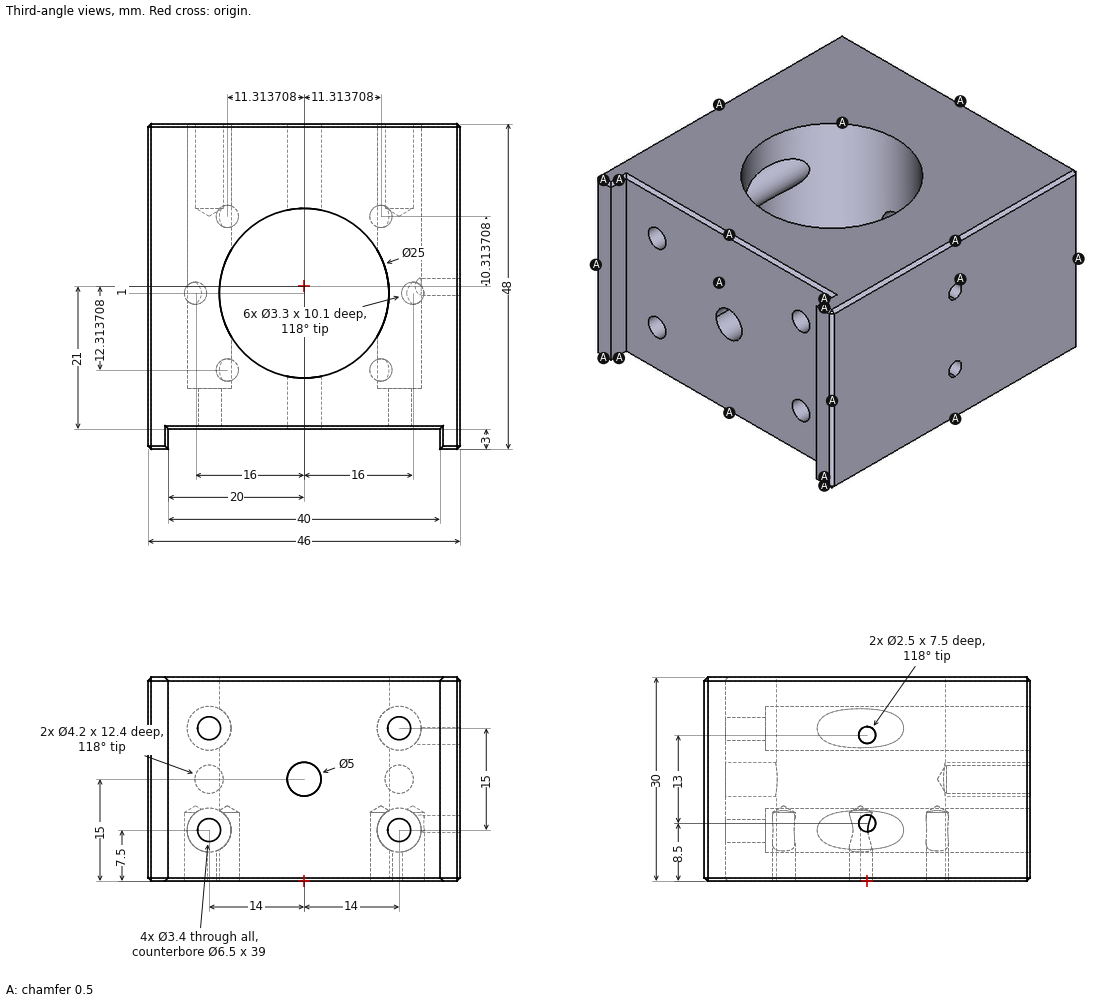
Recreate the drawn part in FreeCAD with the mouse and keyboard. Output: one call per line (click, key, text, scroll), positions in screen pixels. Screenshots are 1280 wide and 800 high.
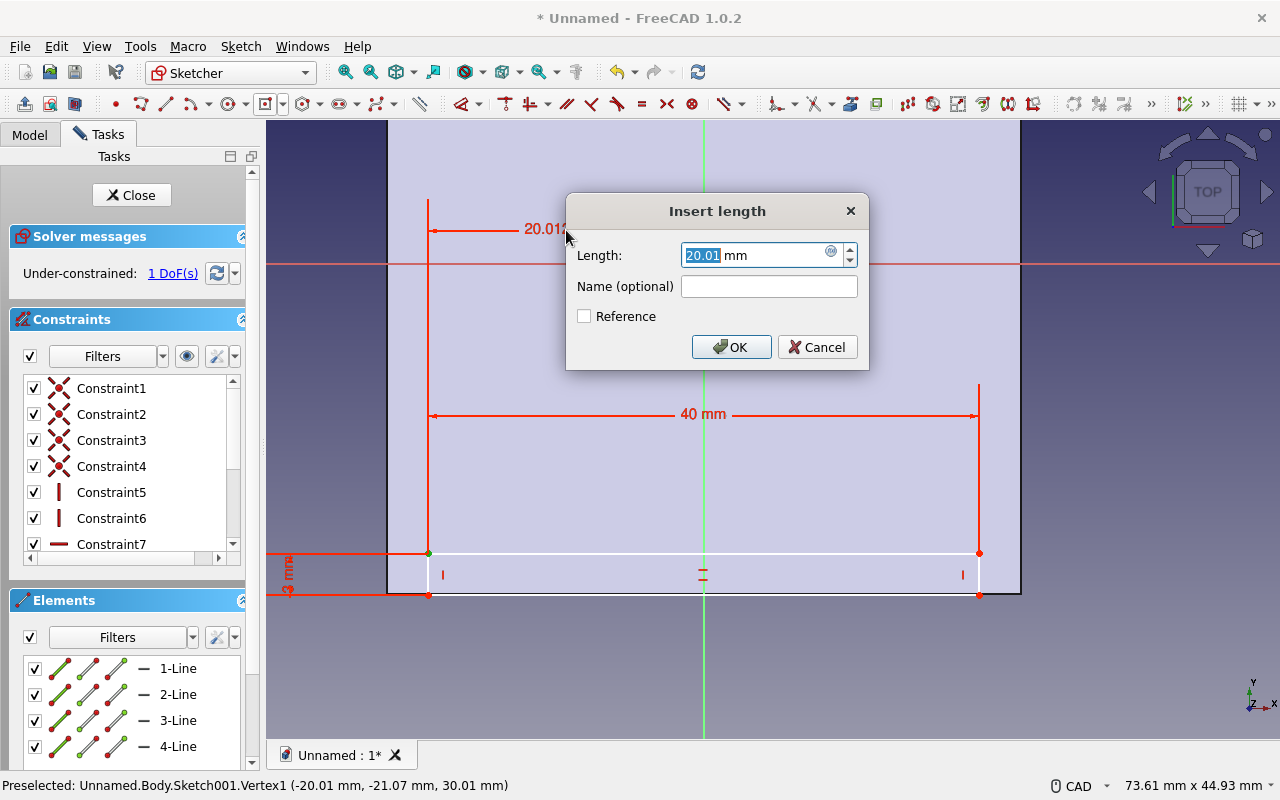
text(20)
key(Return)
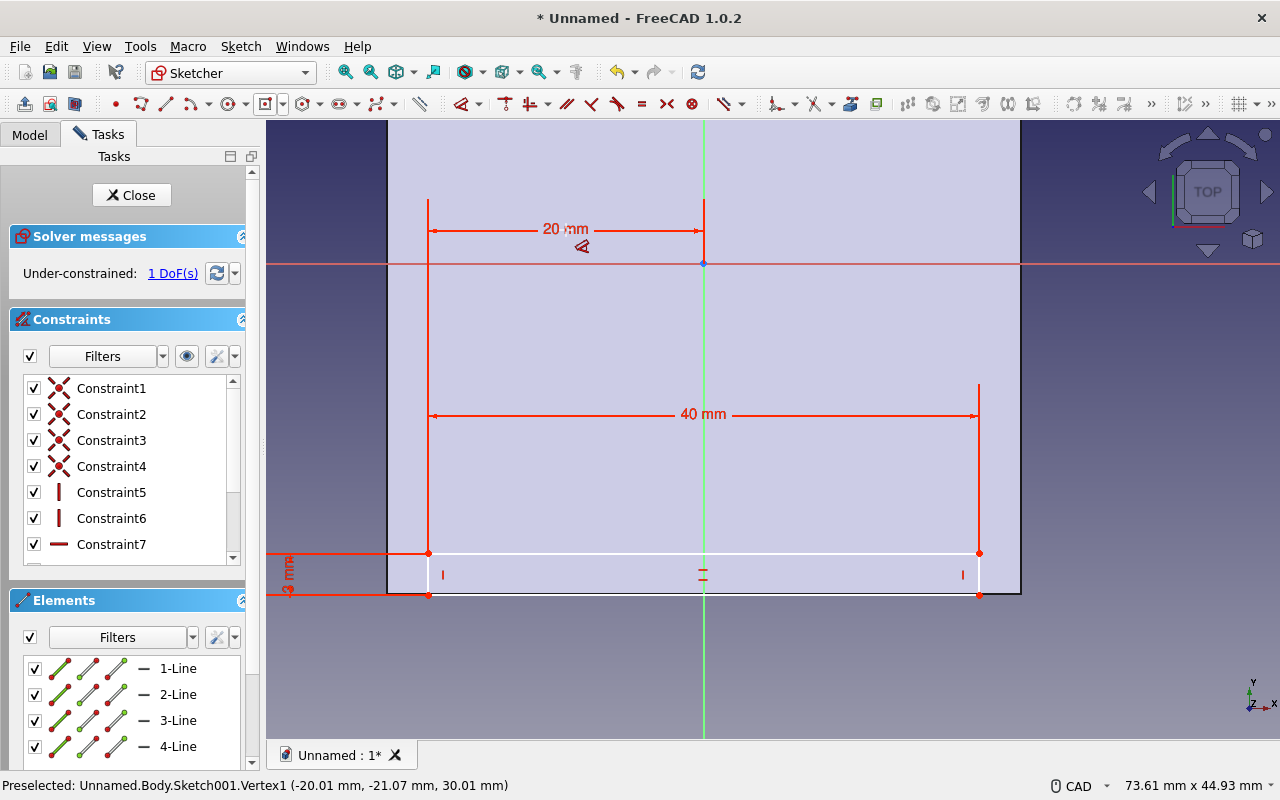
click(428, 554)
click(394, 409)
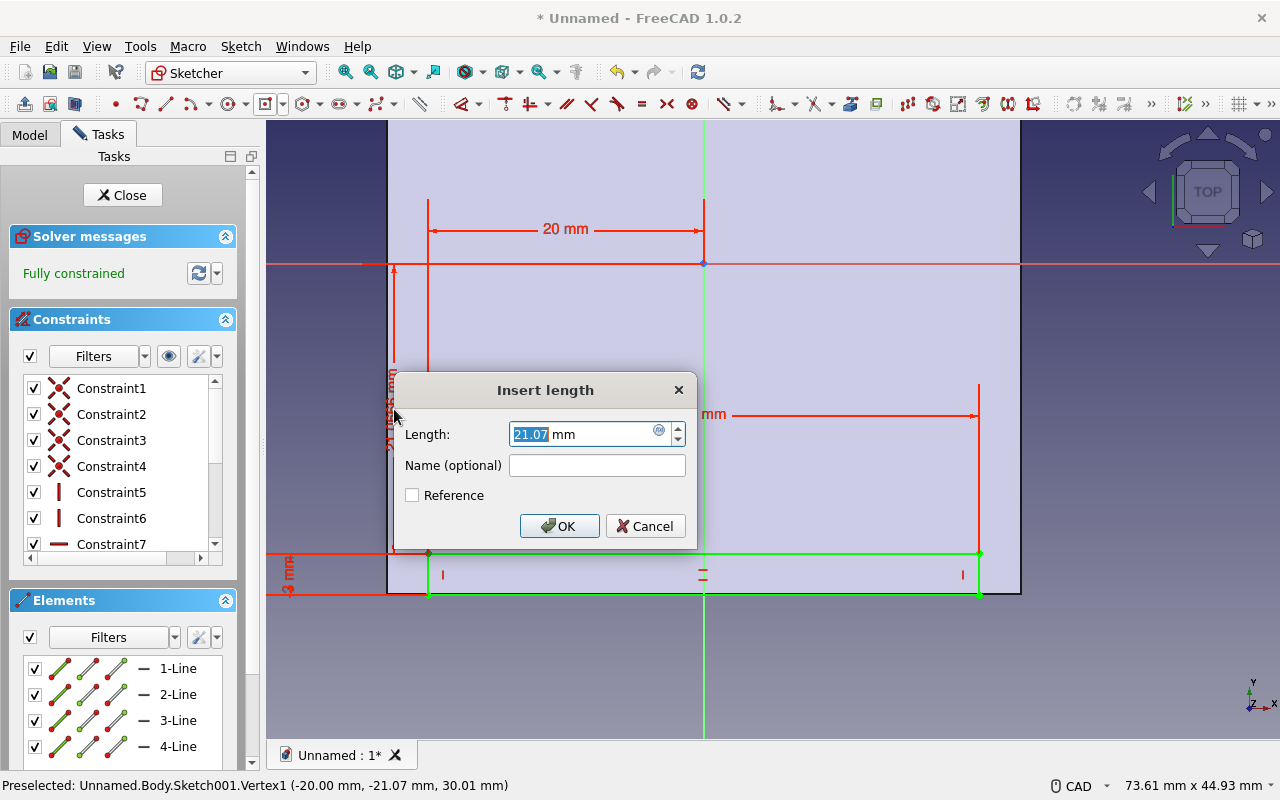
text(21)
key(Return)
key(Escape)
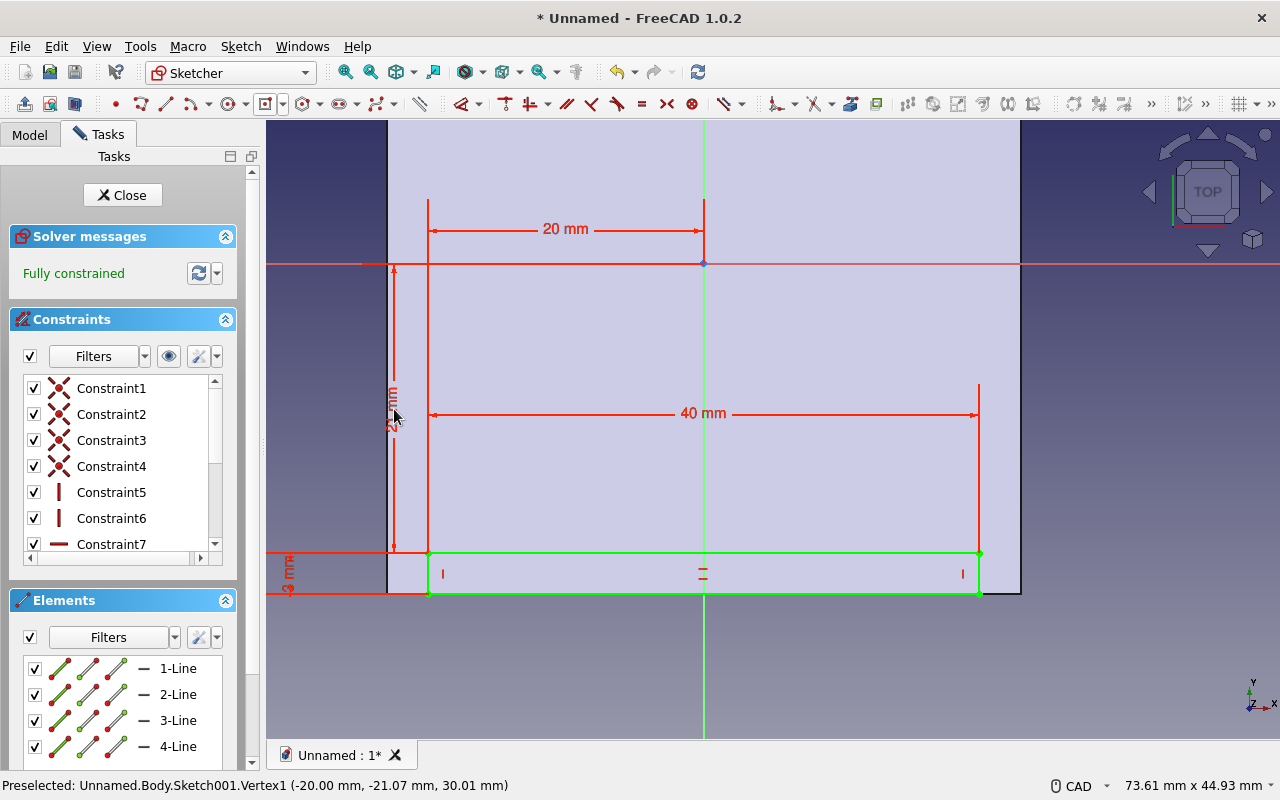
click(123, 195)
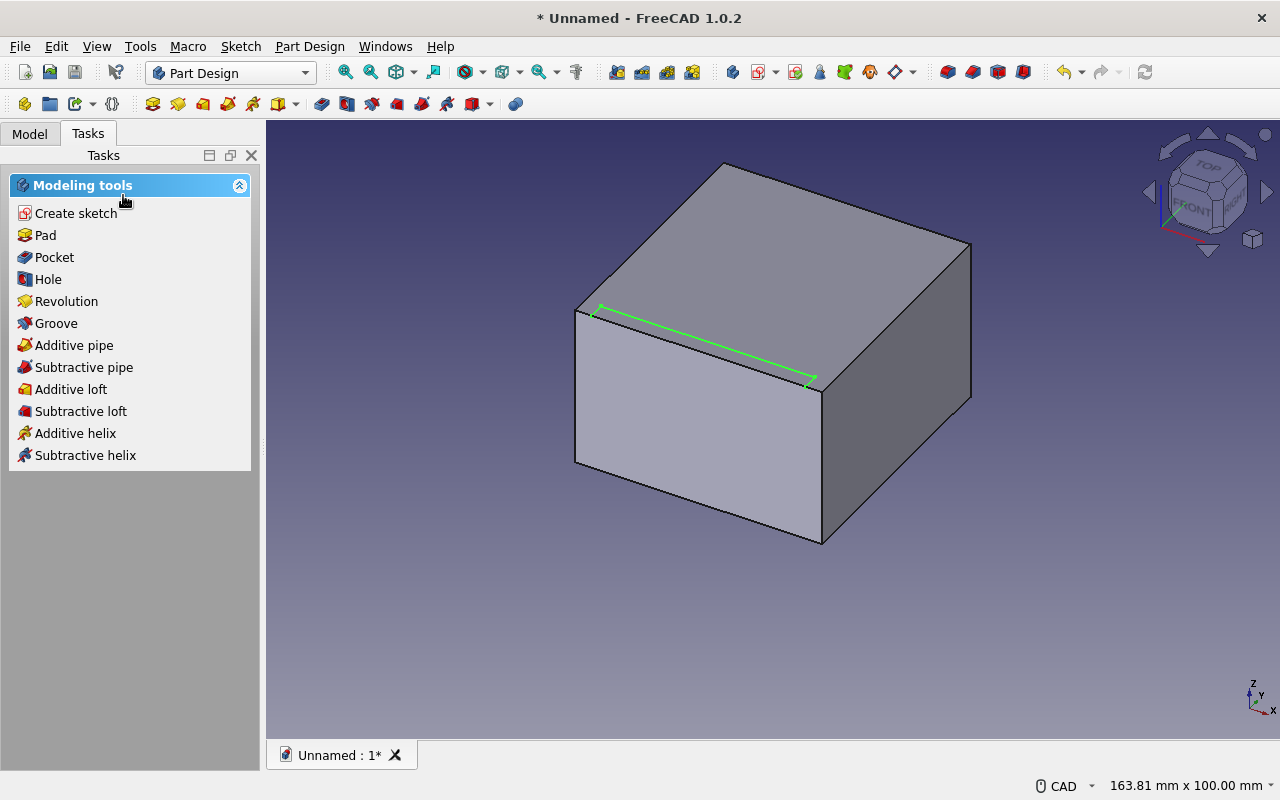
click(322, 104)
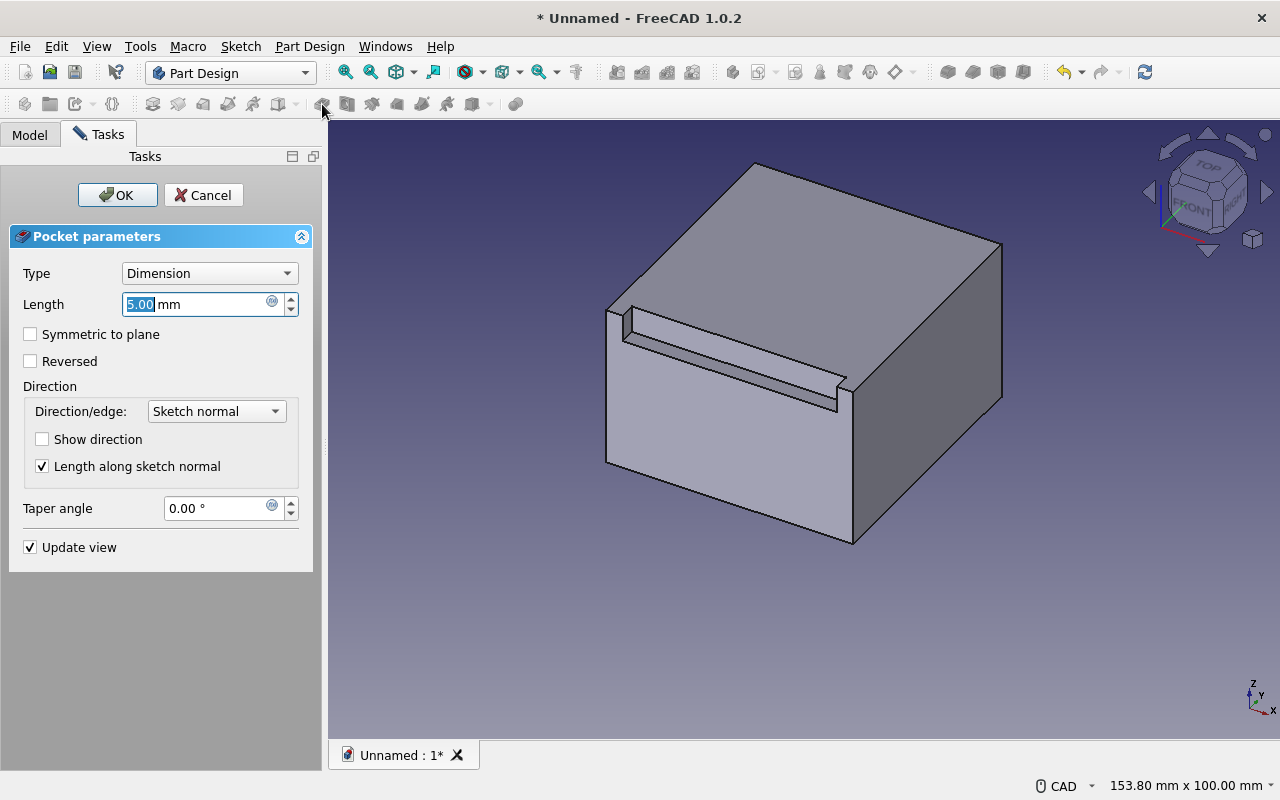
click(210, 274)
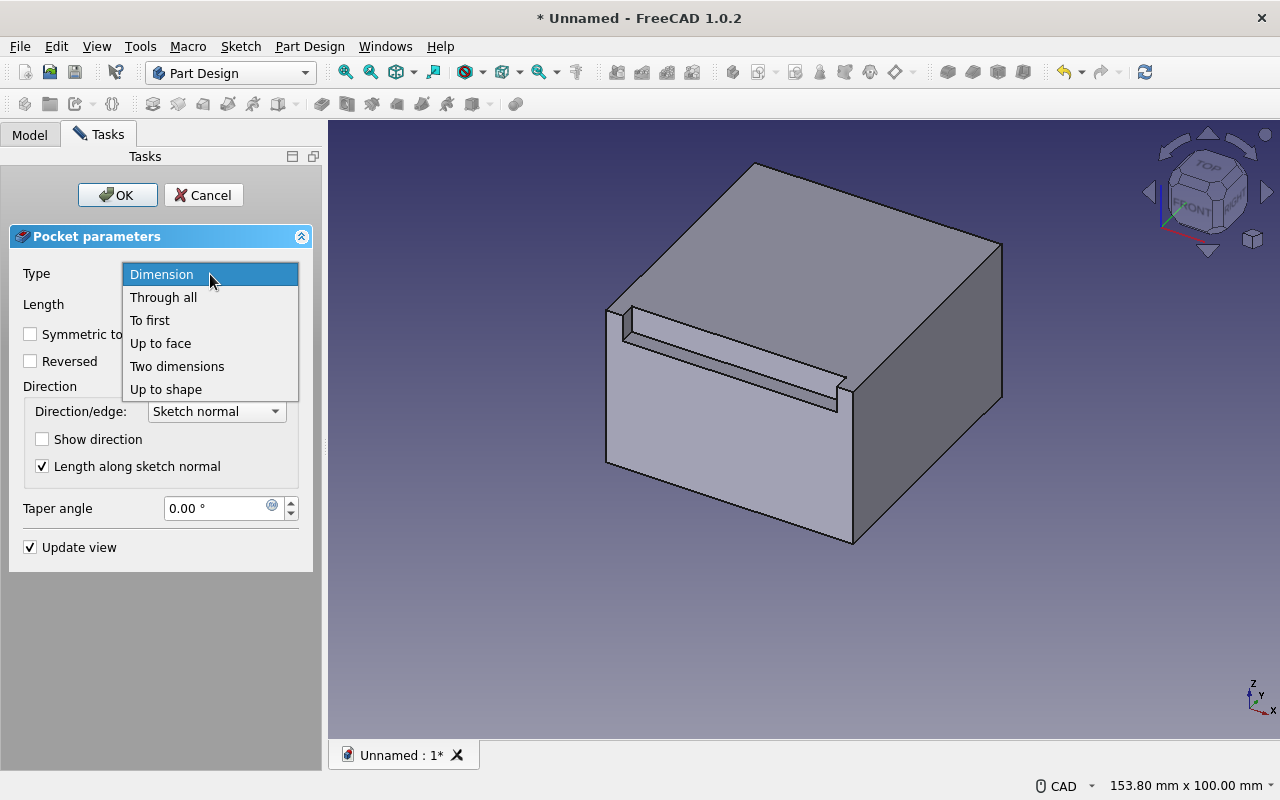
click(208, 298)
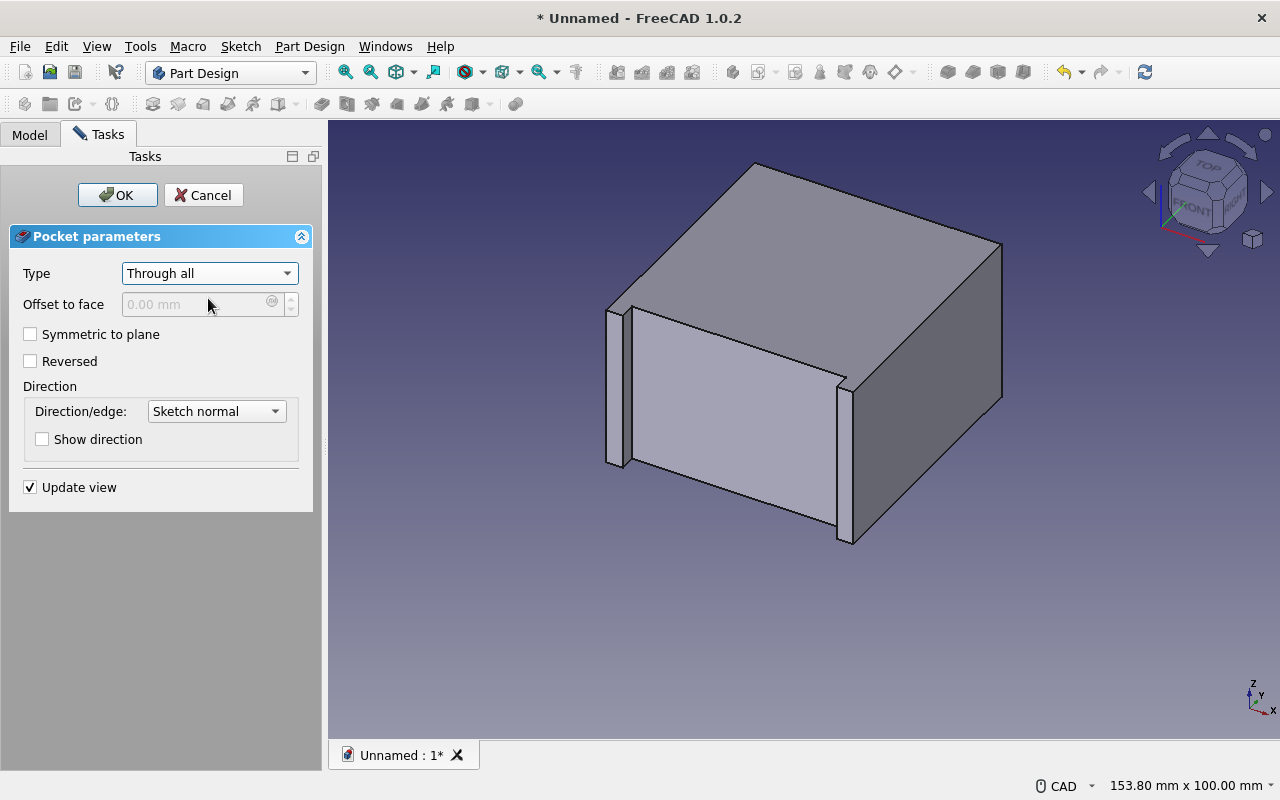
click(118, 195)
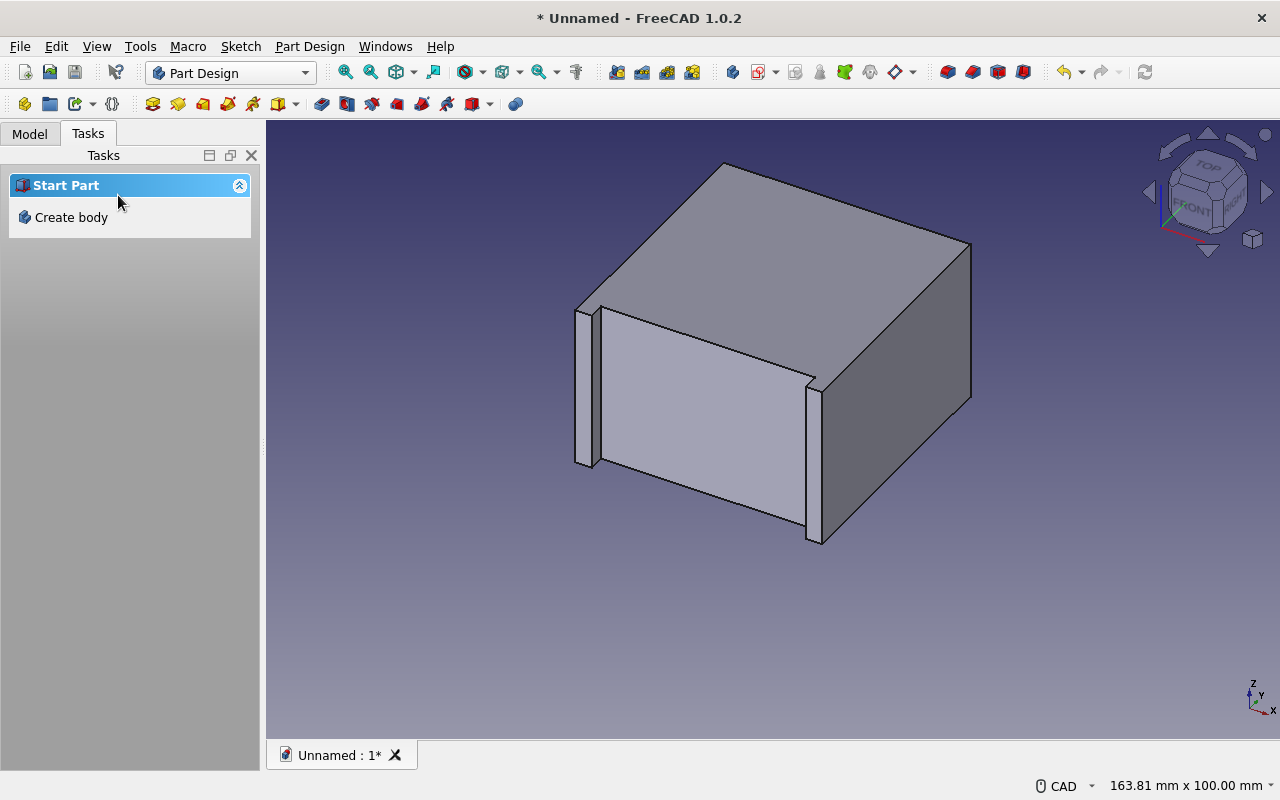
key(4)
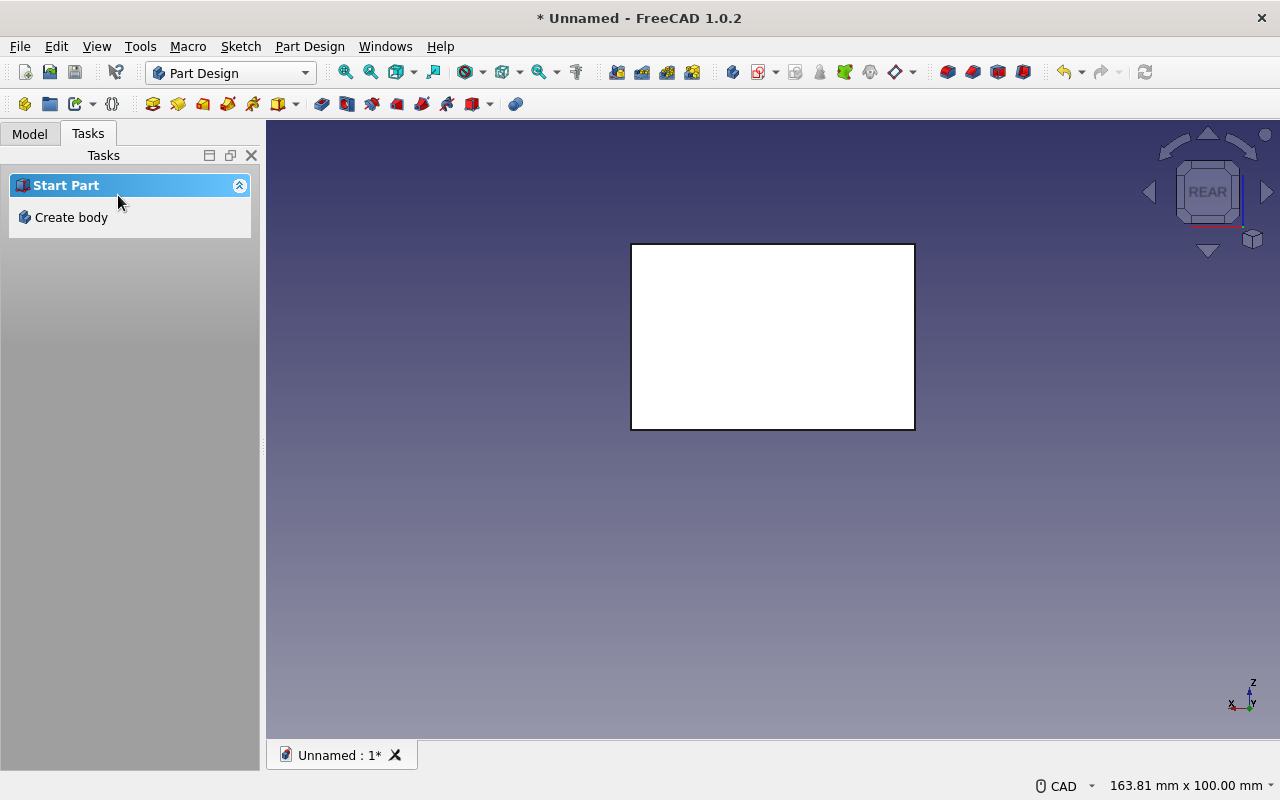
click(346, 72)